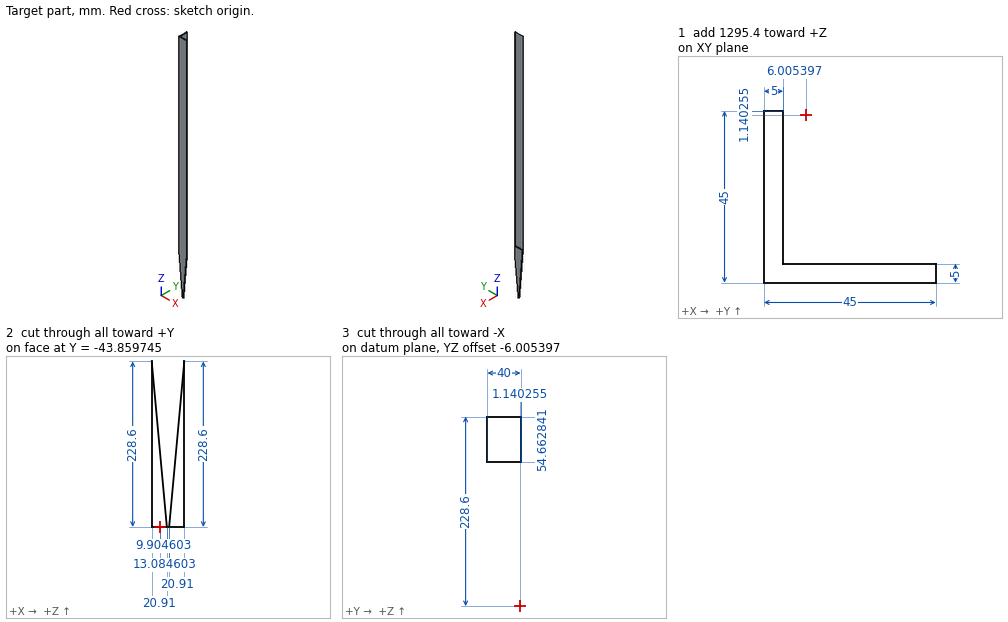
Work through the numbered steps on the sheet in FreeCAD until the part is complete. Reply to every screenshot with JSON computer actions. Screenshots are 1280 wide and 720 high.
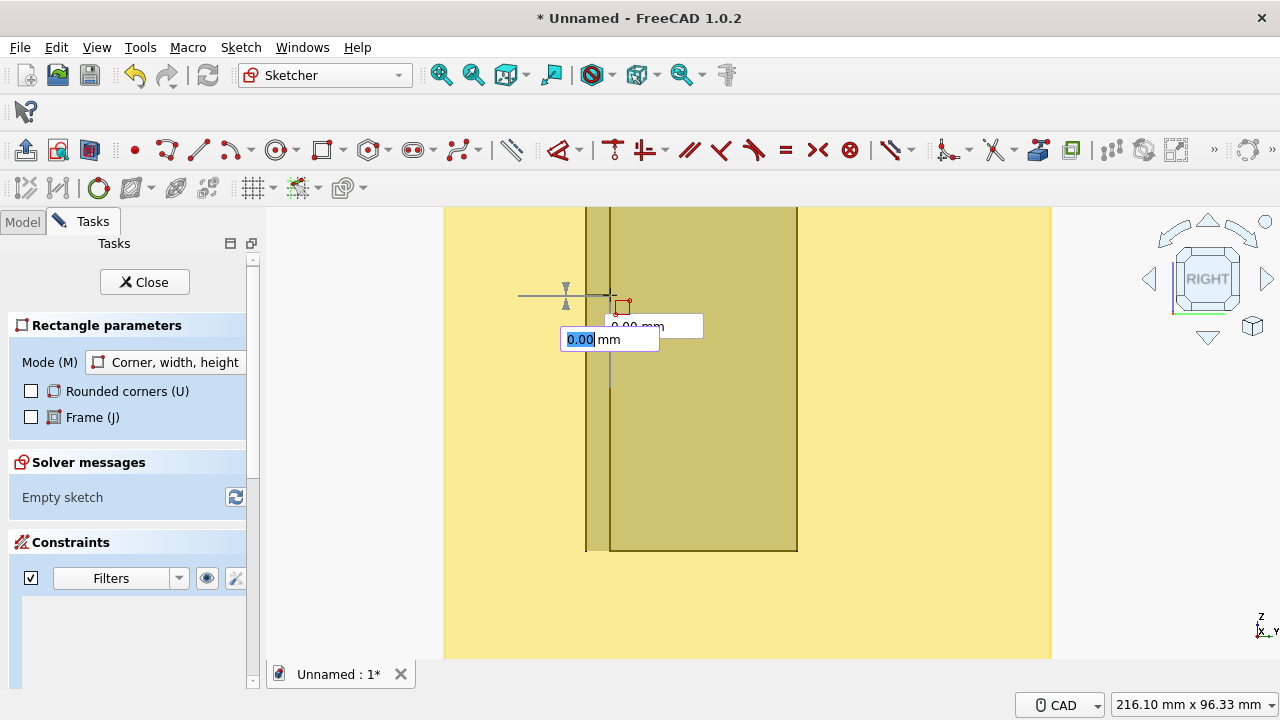
{"action": "scroll", "coordinate": [797, 551], "scroll_direction": "up", "scroll_amount": 6}
{"action": "mouse_move", "coordinate": [797, 550]}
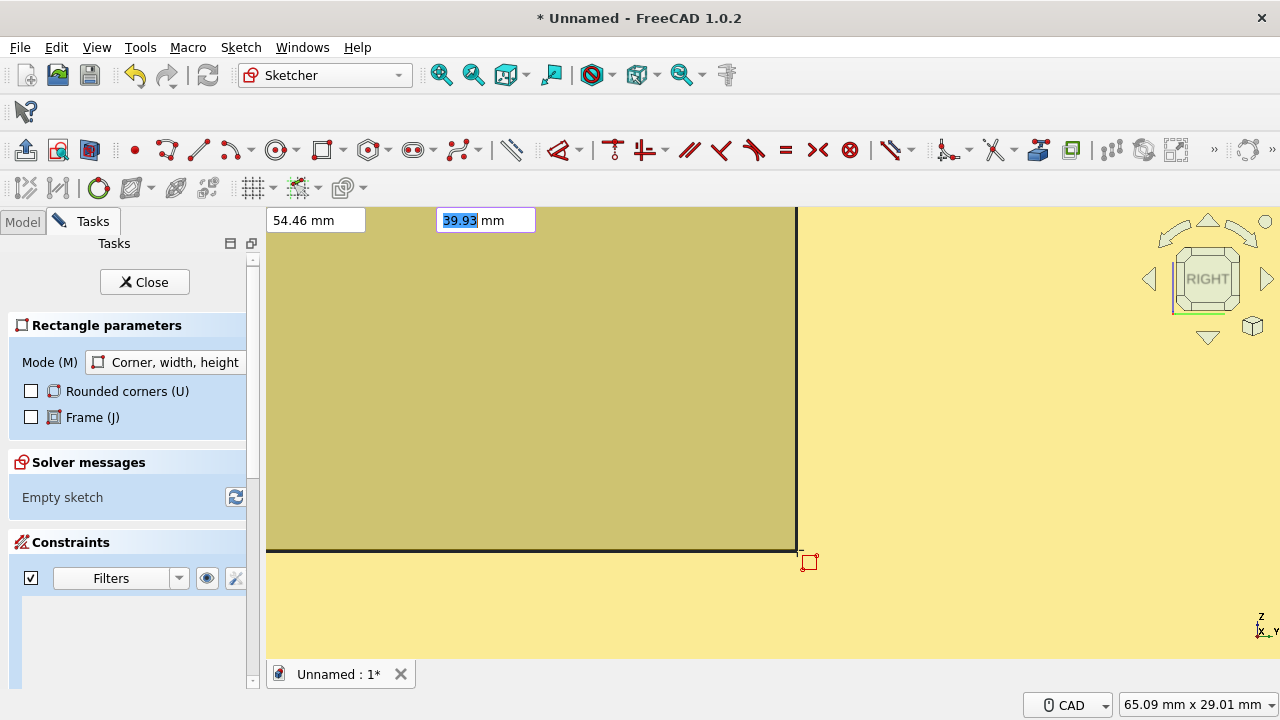
{"action": "type", "text": "40"}
{"action": "key", "text": "Tab"}
{"action": "type", "text": "54.662841"}
{"action": "key", "text": "Return"}
{"action": "key", "text": "Escape"}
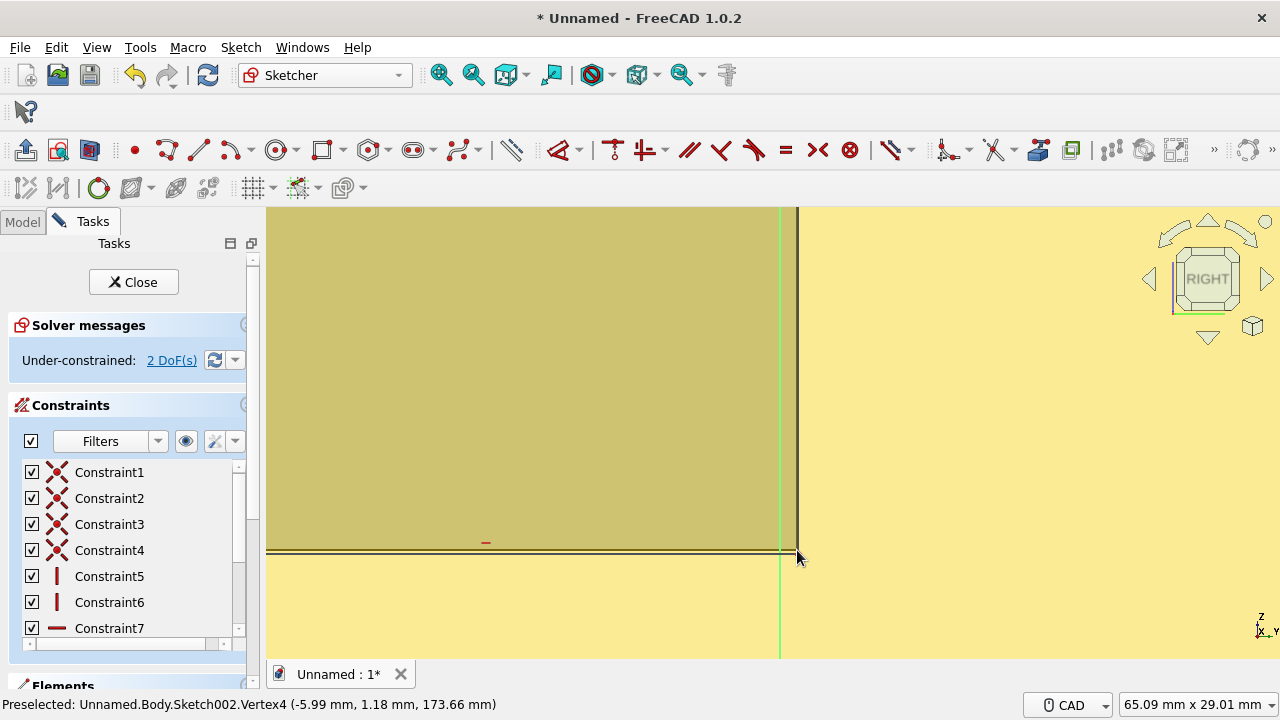
{"action": "left_click", "coordinate": [558, 150]}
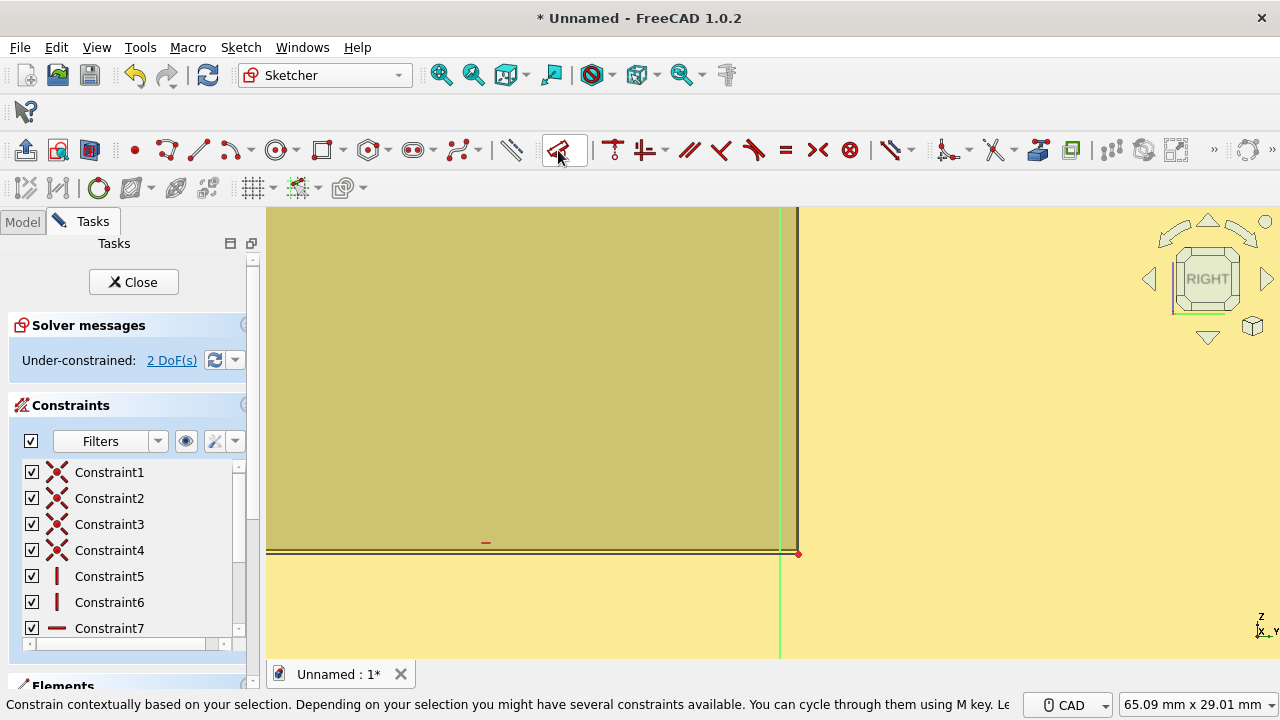
{"action": "scroll", "coordinate": [799, 566], "scroll_direction": "down", "scroll_amount": 6}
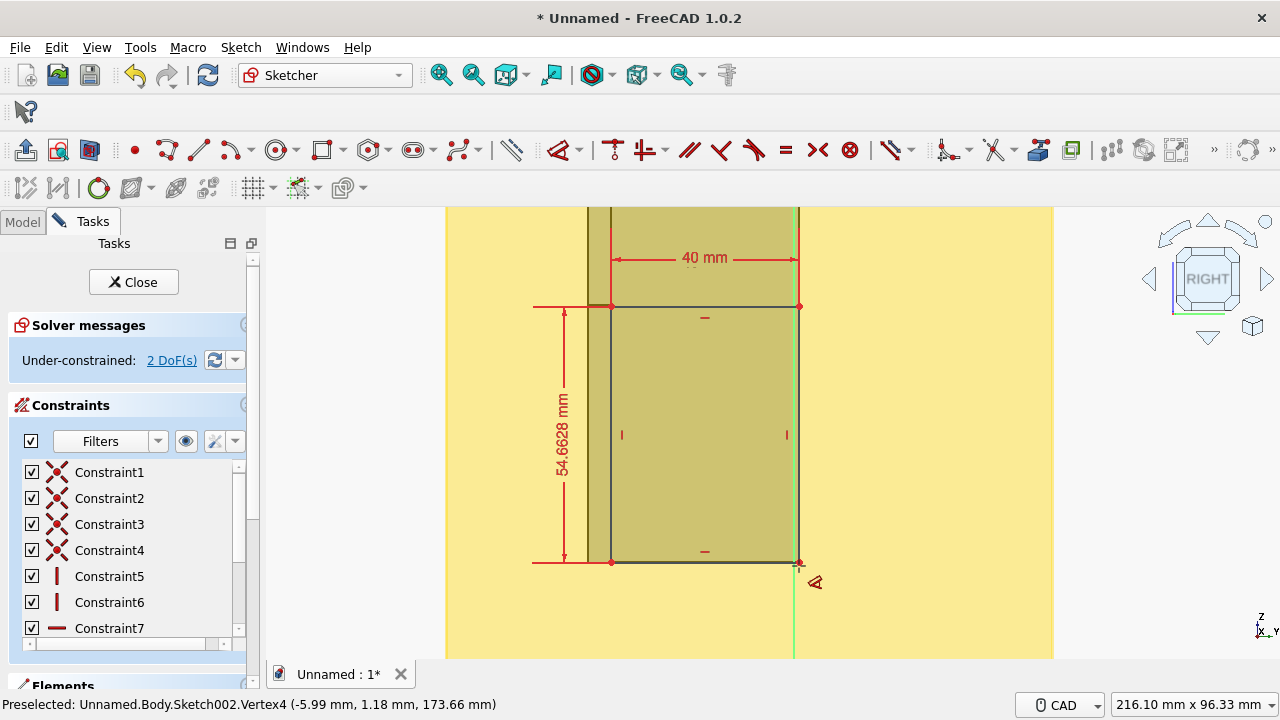
{"action": "left_click", "coordinate": [611, 307]}
{"action": "left_click", "coordinate": [577, 469]}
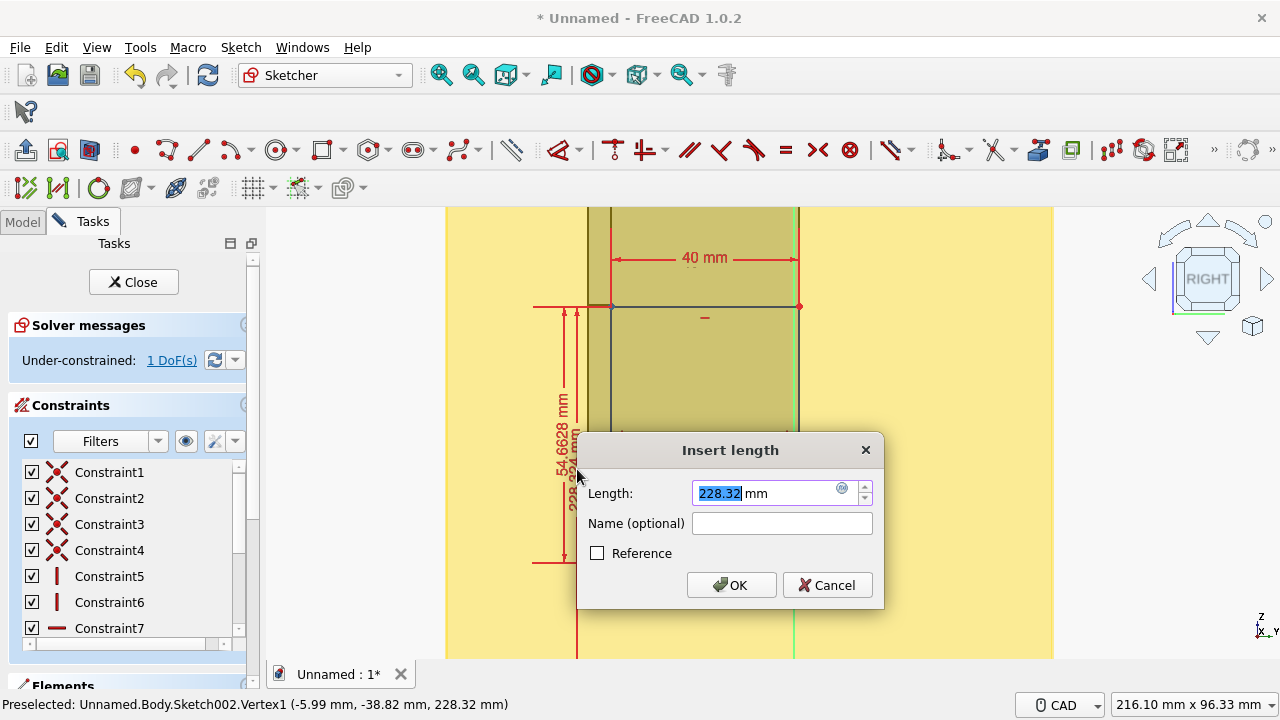
{"action": "type", "text": "228.6"}
{"action": "key", "text": "Return"}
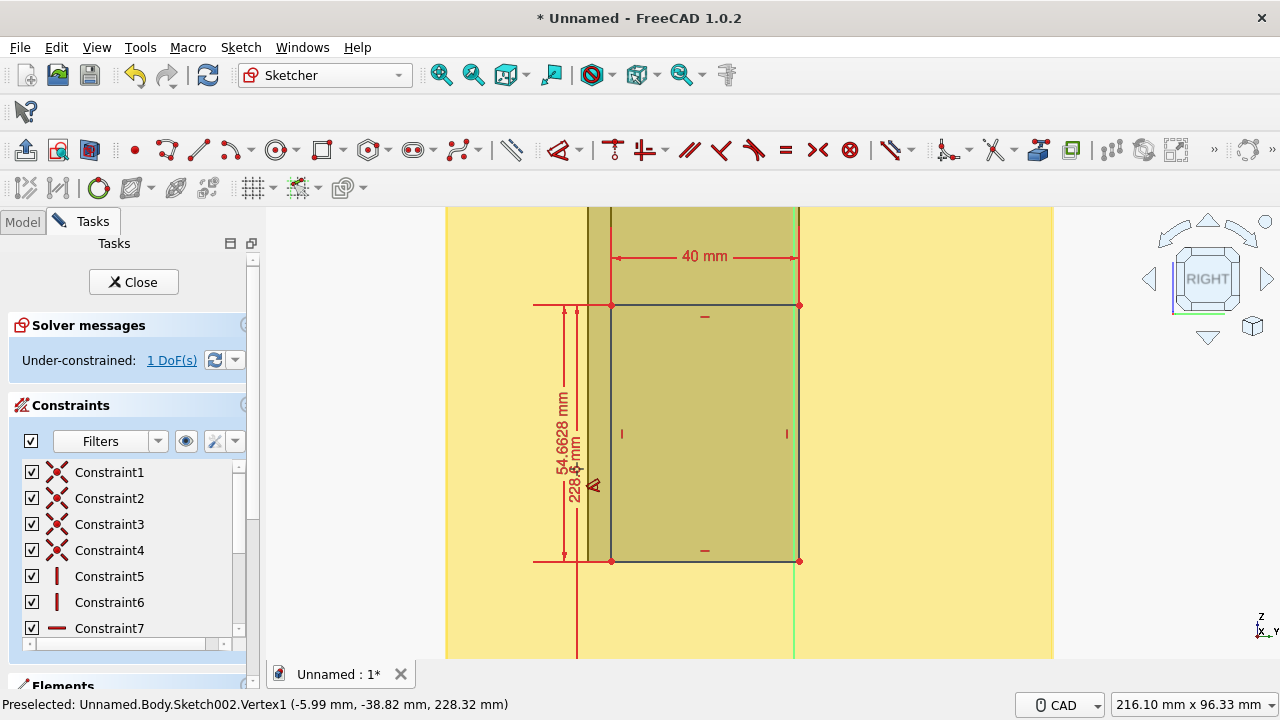
{"action": "scroll", "coordinate": [799, 562], "scroll_direction": "up", "scroll_amount": 11}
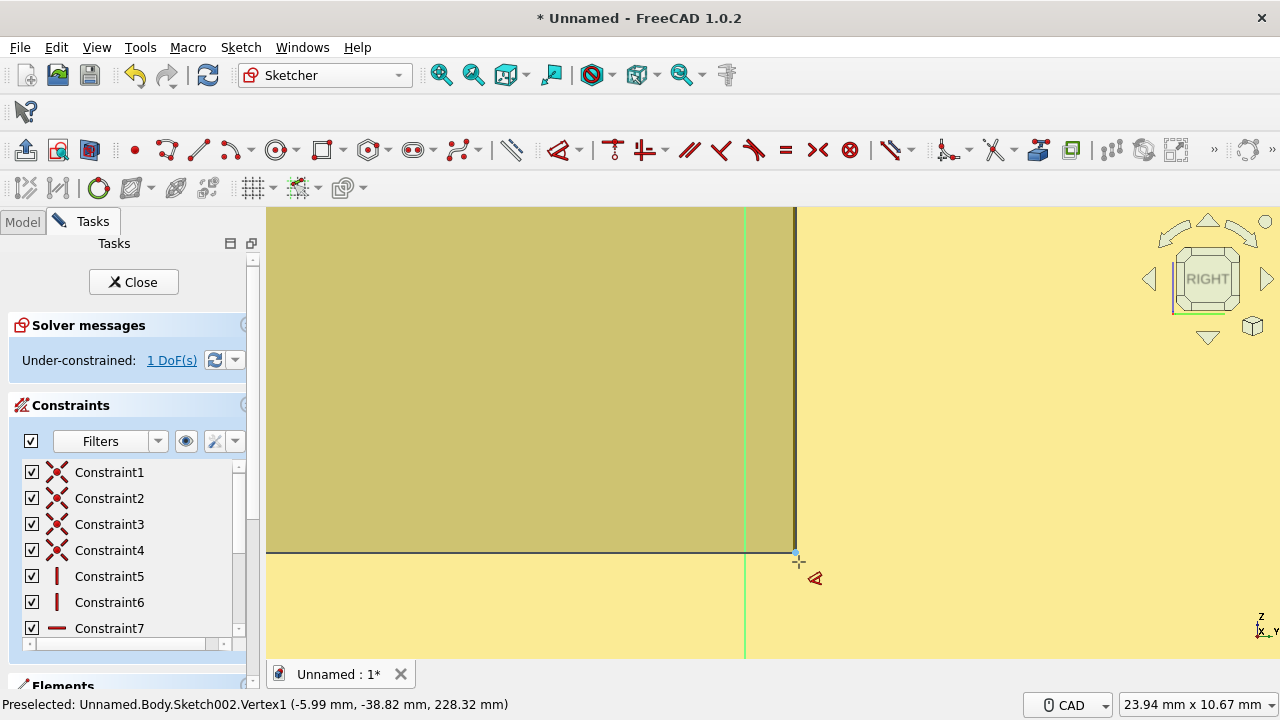
{"action": "left_click", "coordinate": [796, 553]}
{"action": "left_click", "coordinate": [770, 519]}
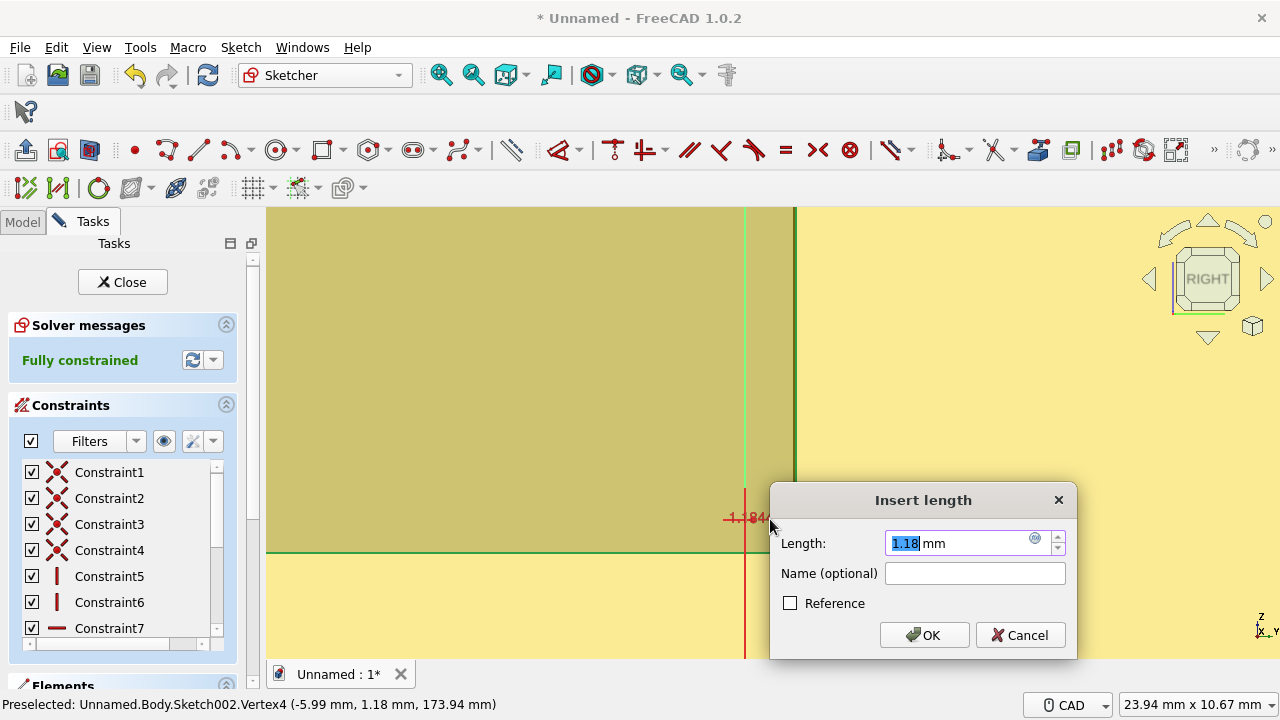
{"action": "type", "text": "1.140255"}
{"action": "key", "text": "Return"}
{"action": "key", "text": "Escape"}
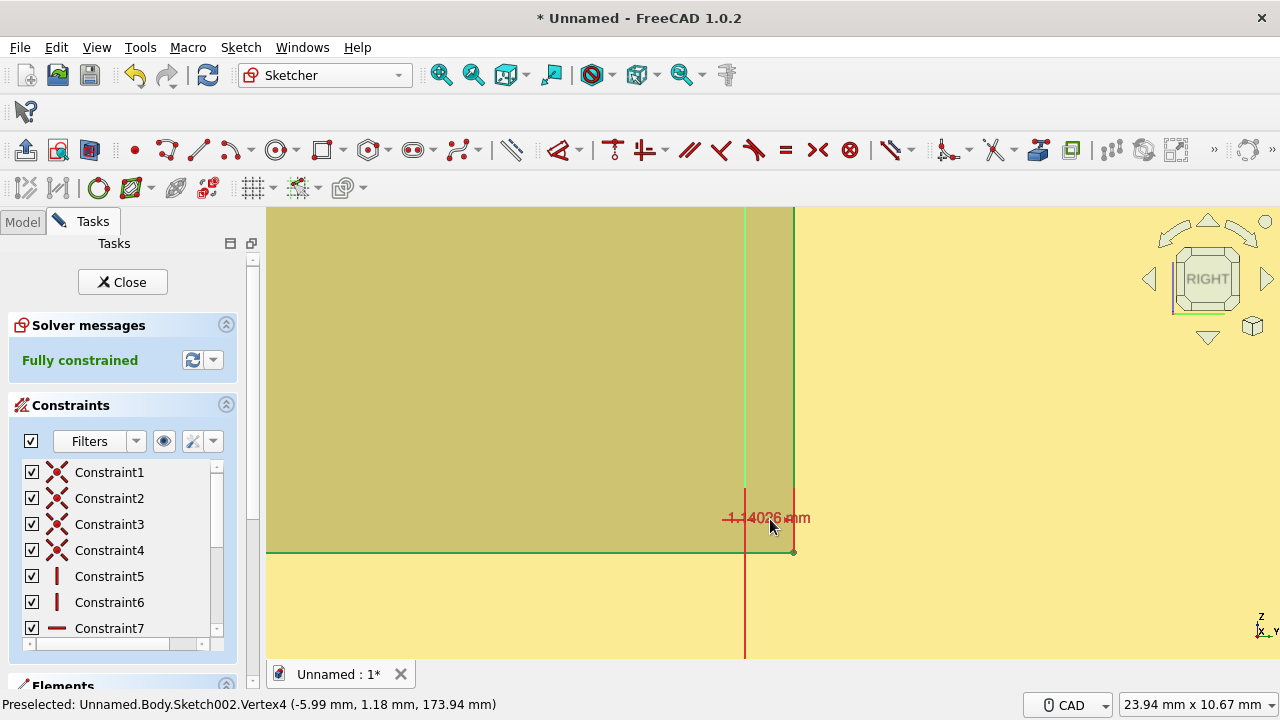
{"action": "left_click", "coordinate": [123, 282]}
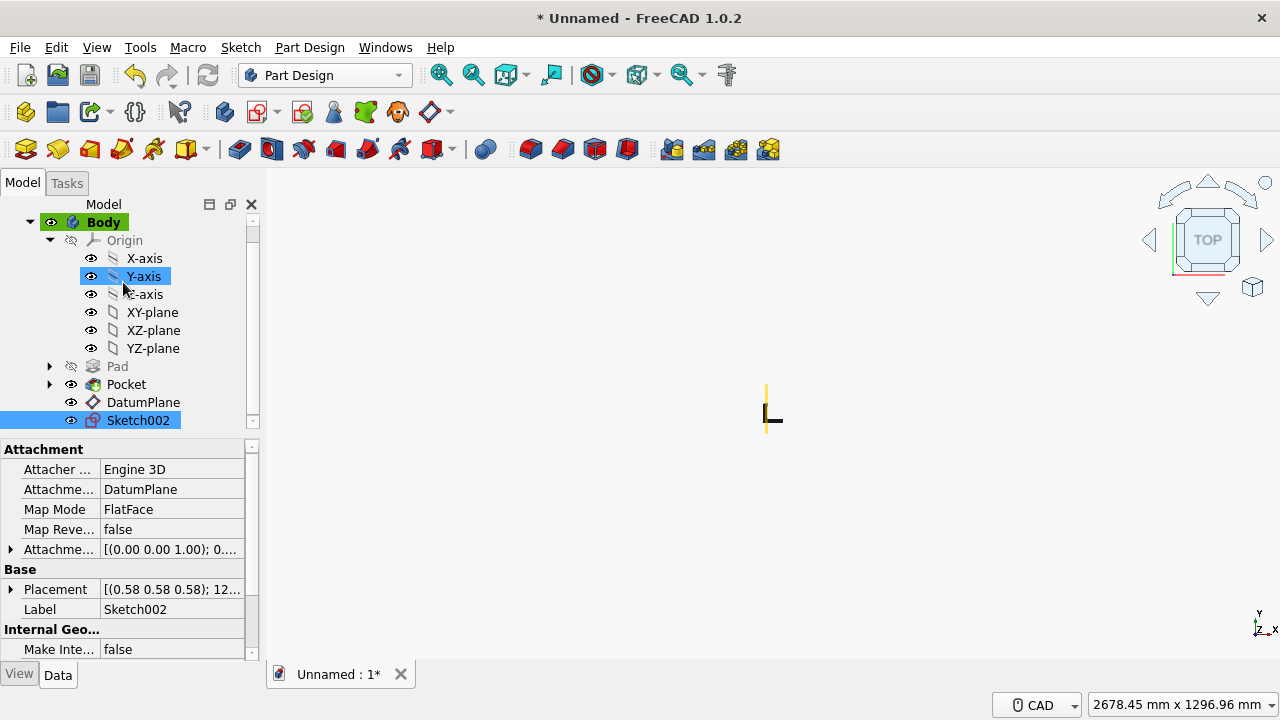
{"action": "left_click", "coordinate": [240, 150]}